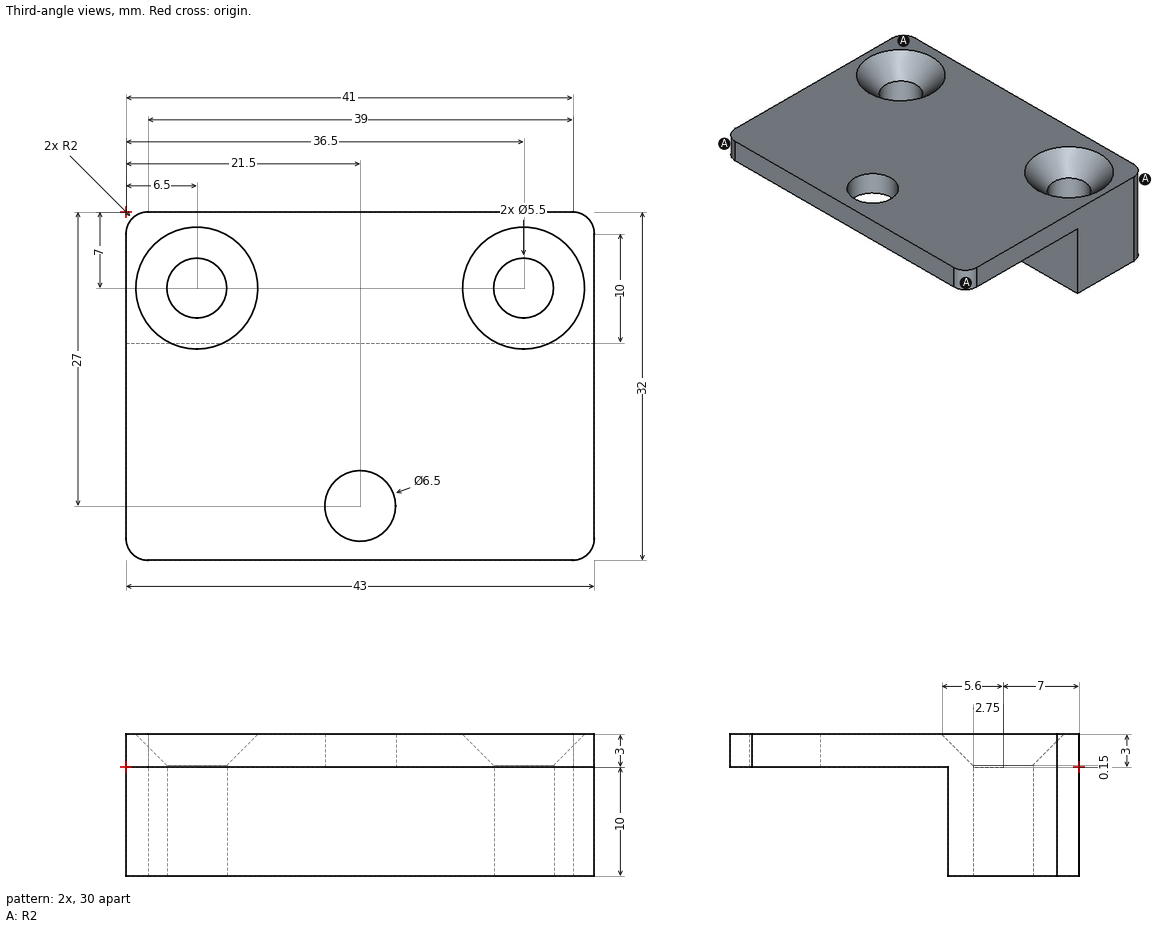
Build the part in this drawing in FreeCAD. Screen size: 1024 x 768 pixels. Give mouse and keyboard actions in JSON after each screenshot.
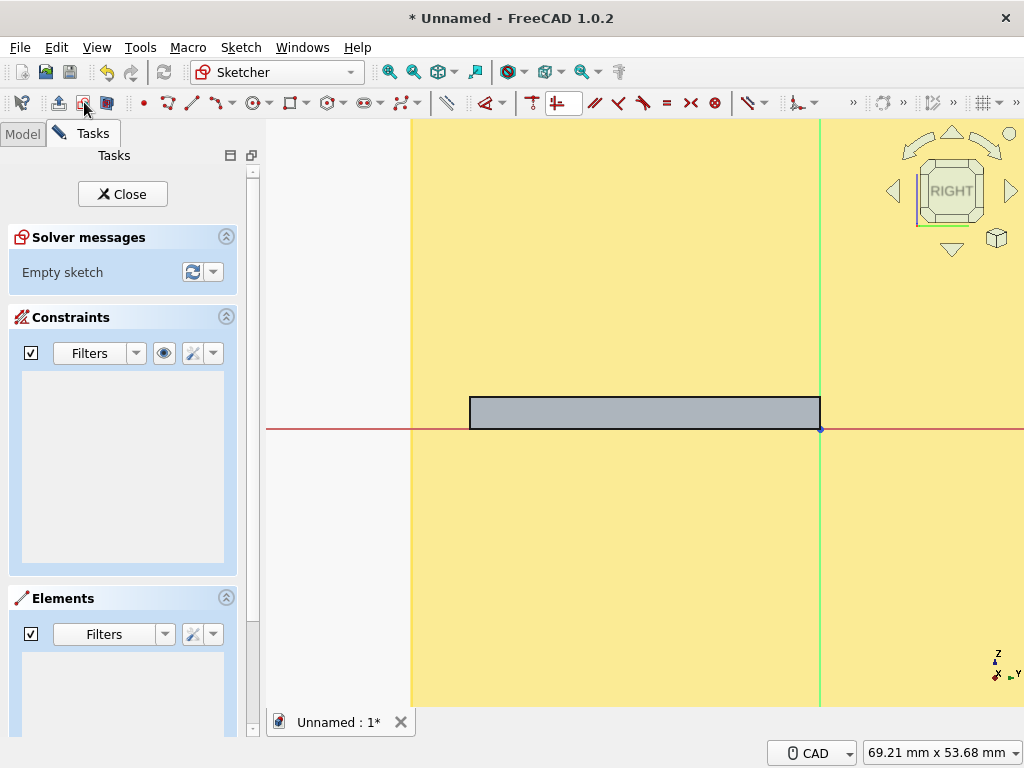
{"action": "key", "text": "q s"}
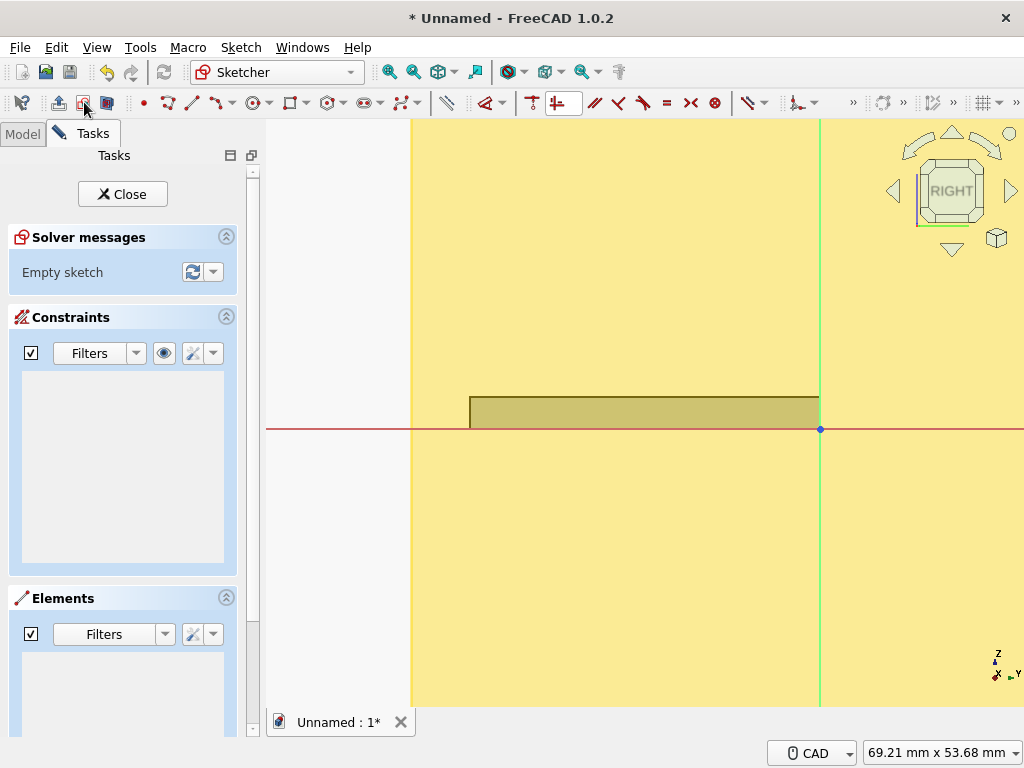
{"action": "scroll", "coordinate": [853, 423], "scroll_direction": "up", "scroll_amount": 5}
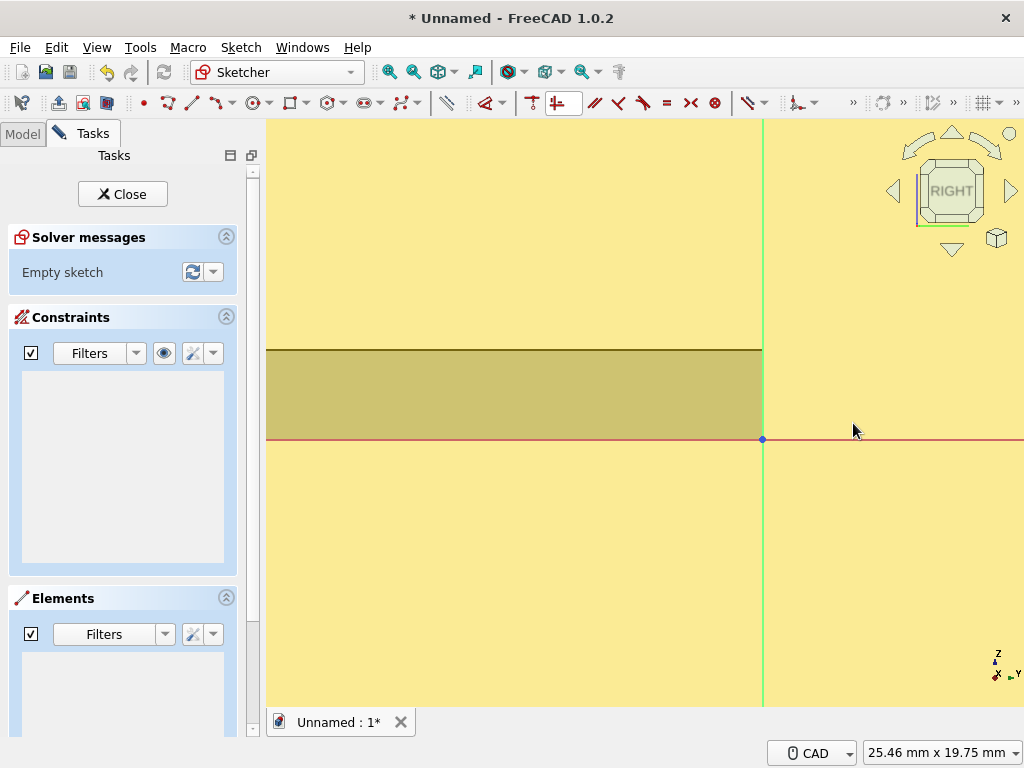
{"action": "left_click", "coordinate": [168, 104]}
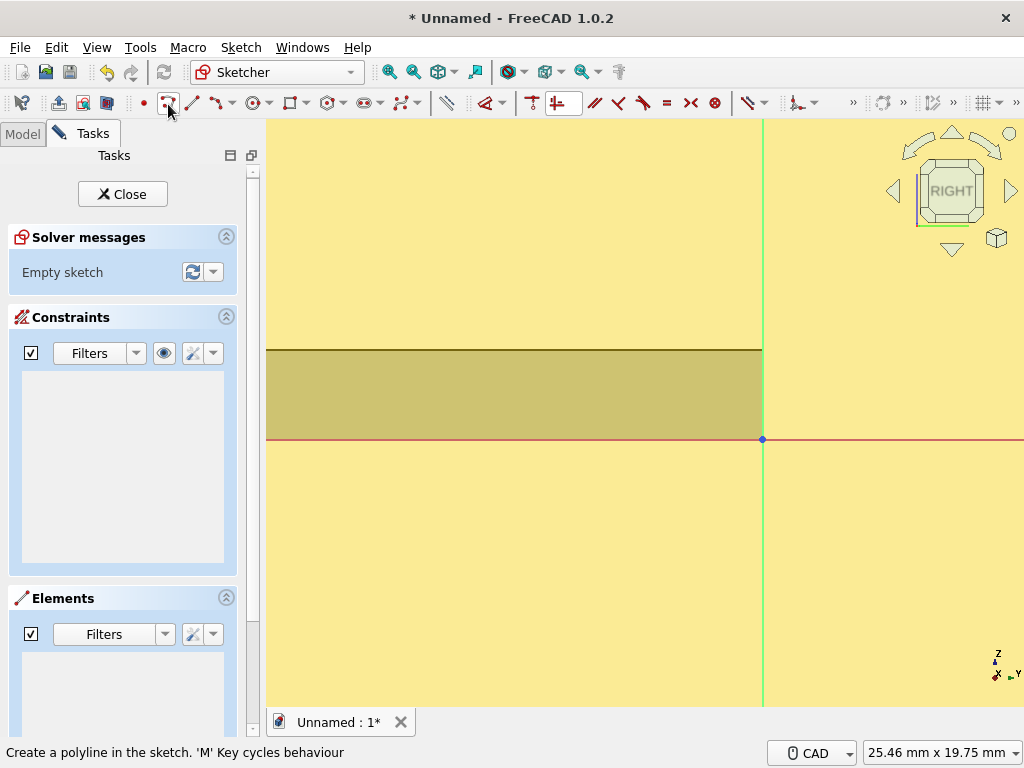
{"action": "left_click", "coordinate": [554, 440]}
{"action": "left_click", "coordinate": [554, 350]}
{"action": "left_click", "coordinate": [387, 350]}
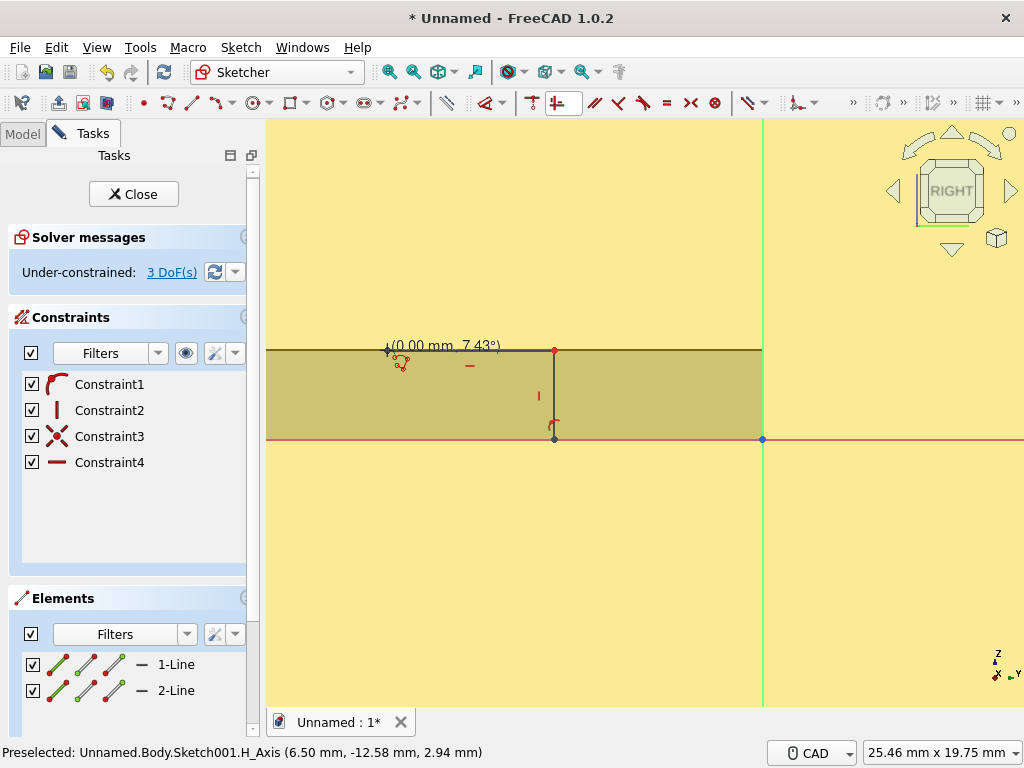
{"action": "scroll", "coordinate": [472, 435], "scroll_direction": "up", "scroll_amount": 7}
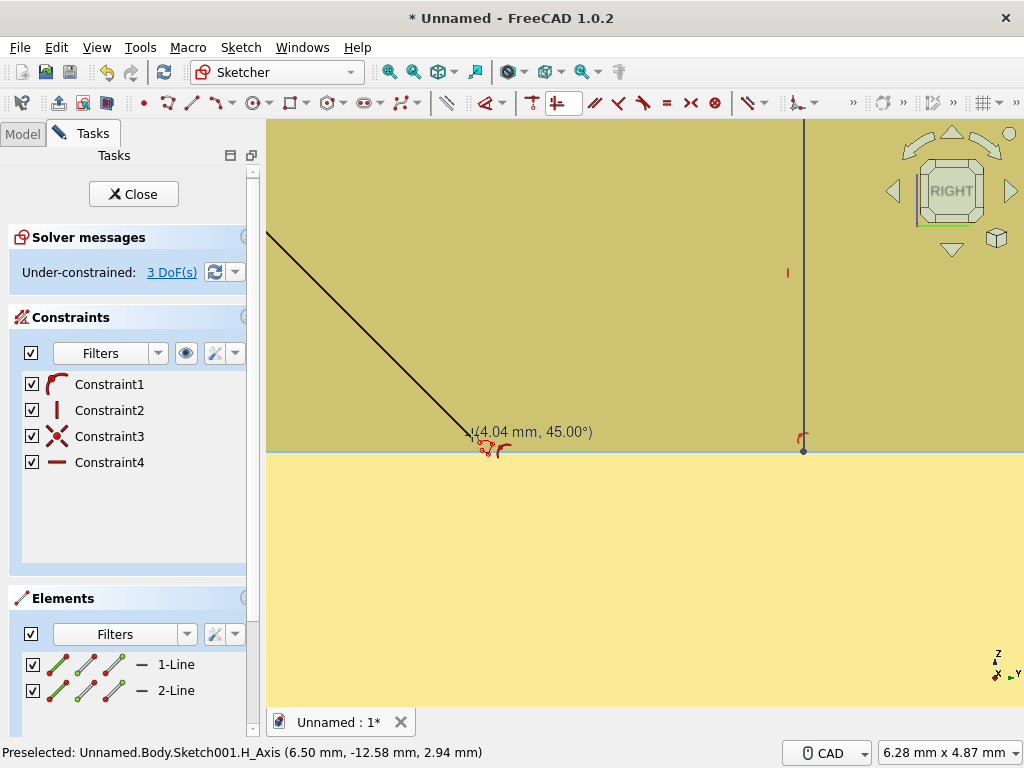
{"action": "left_click", "coordinate": [473, 434]}
{"action": "left_click", "coordinate": [473, 443]}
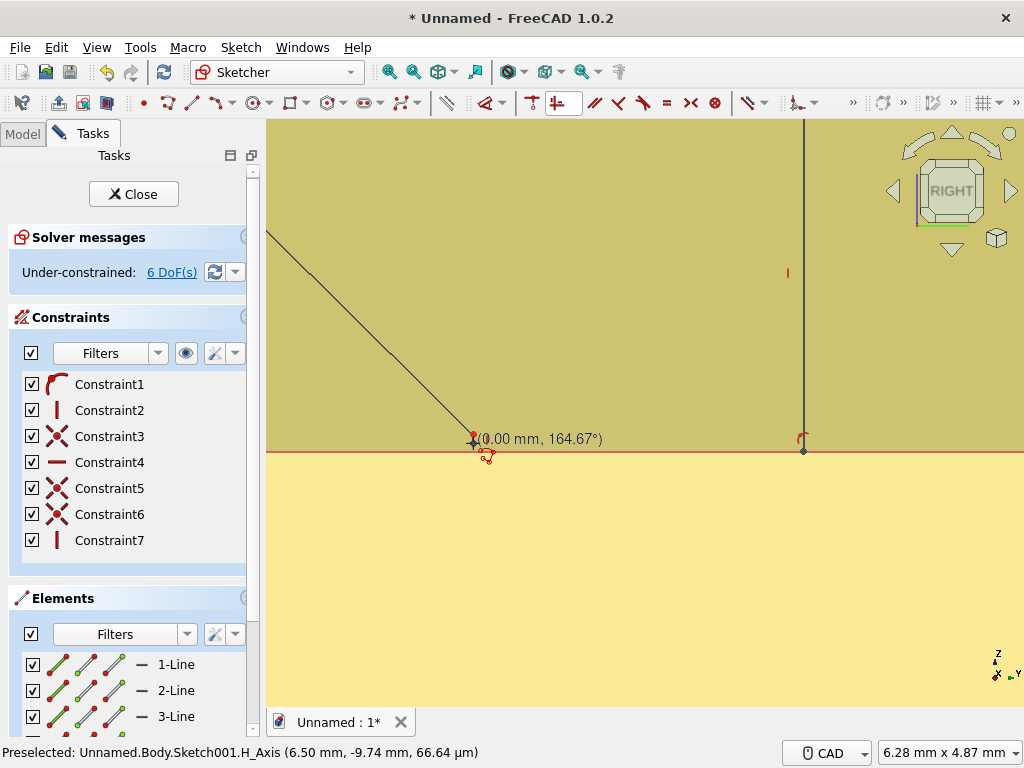
{"action": "scroll", "coordinate": [474, 436], "scroll_direction": "down", "scroll_amount": 7}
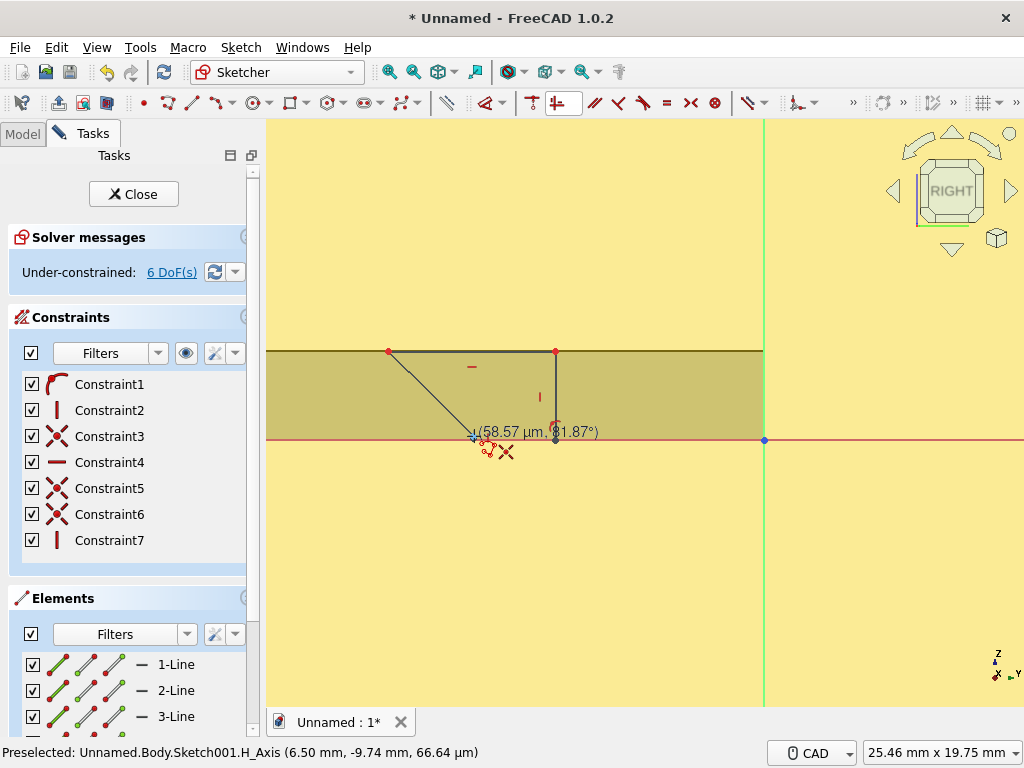
{"action": "left_click", "coordinate": [556, 440]}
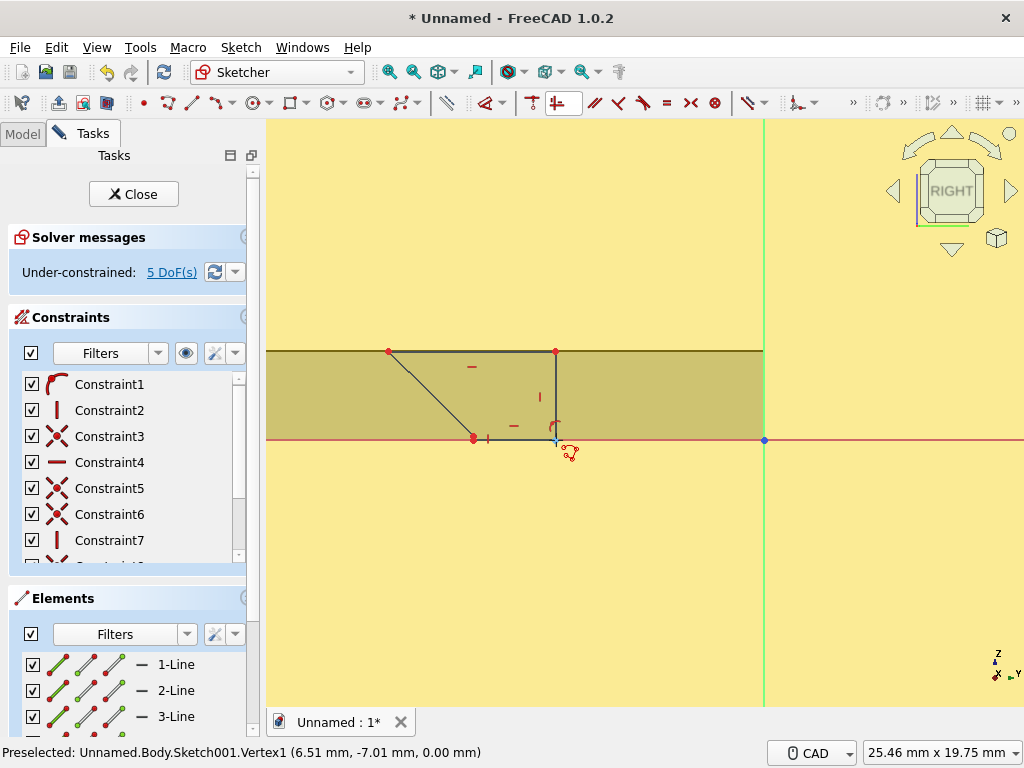
{"action": "key", "text": "g l"}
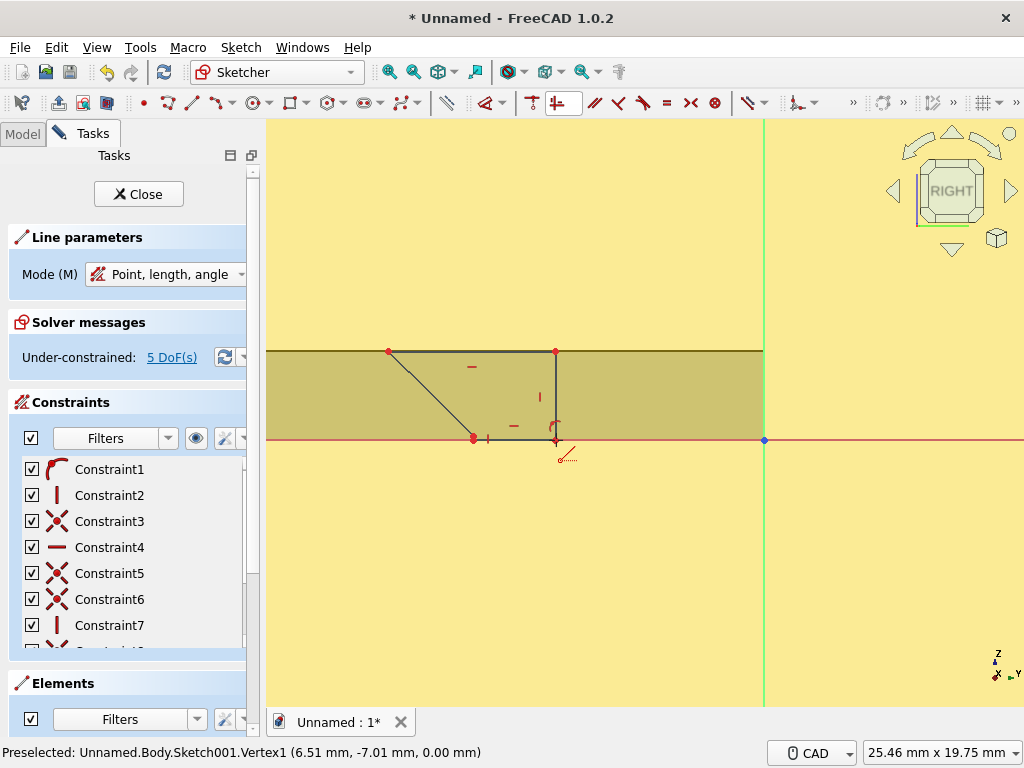
{"action": "scroll", "coordinate": [556, 449], "scroll_direction": "up", "scroll_amount": 3}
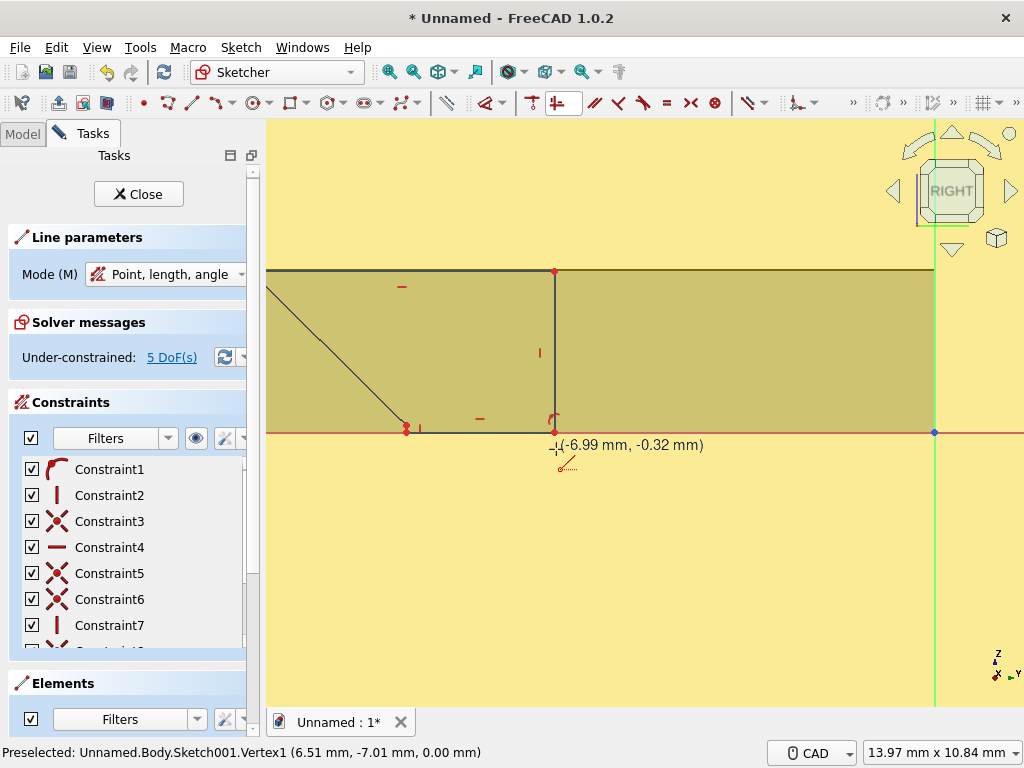
{"action": "left_click", "coordinate": [555, 449]}
{"action": "left_click", "coordinate": [555, 498]}
{"action": "key", "text": "Escape"}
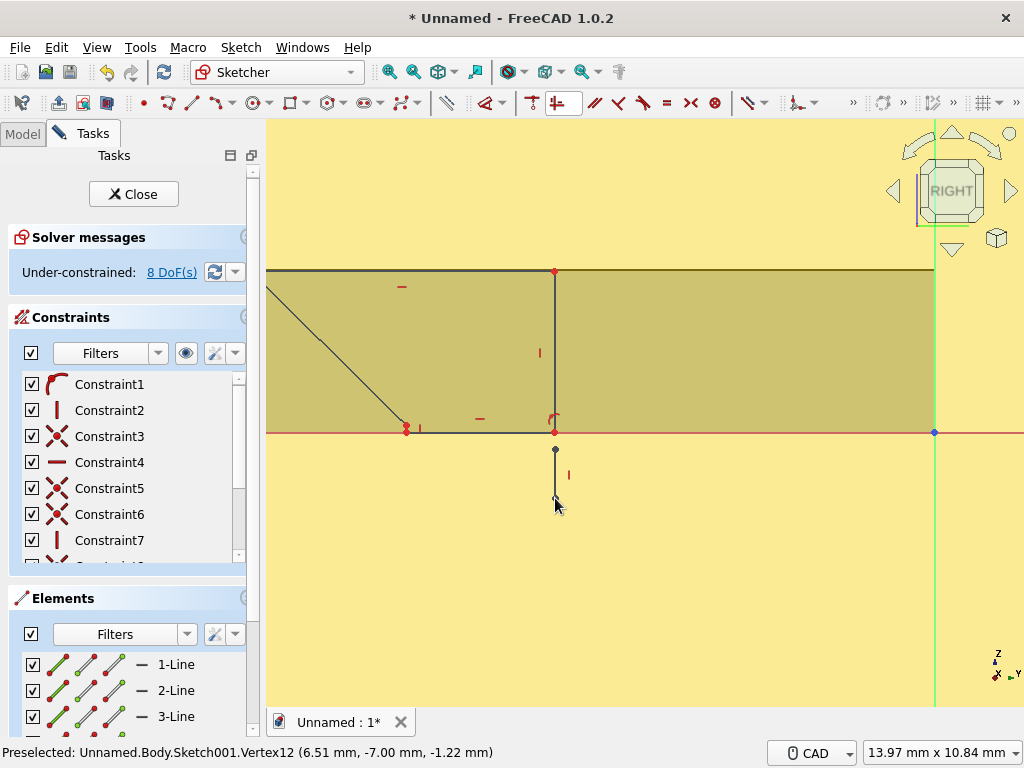
{"action": "left_click", "coordinate": [555, 465]}